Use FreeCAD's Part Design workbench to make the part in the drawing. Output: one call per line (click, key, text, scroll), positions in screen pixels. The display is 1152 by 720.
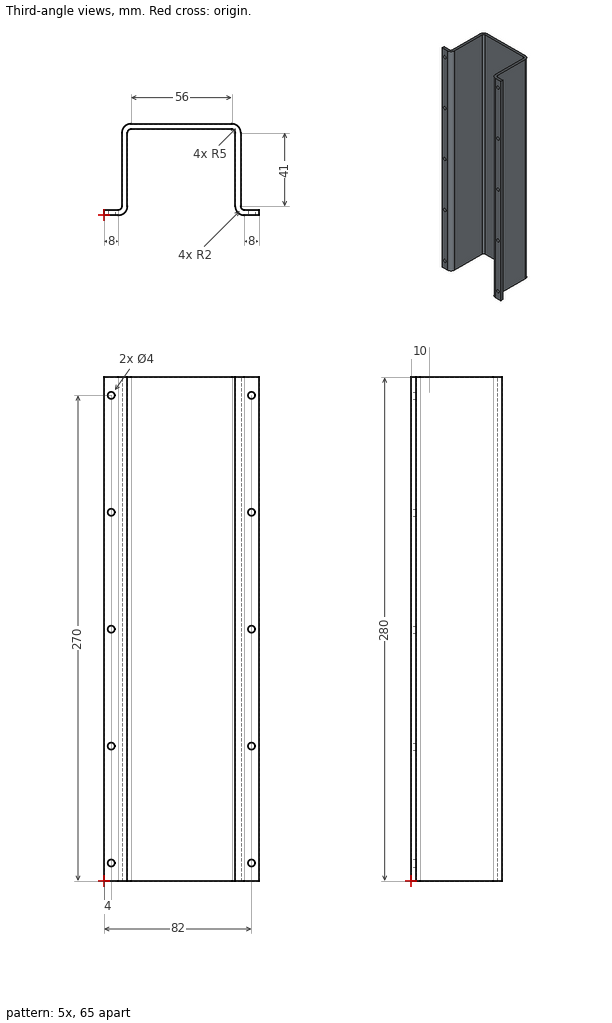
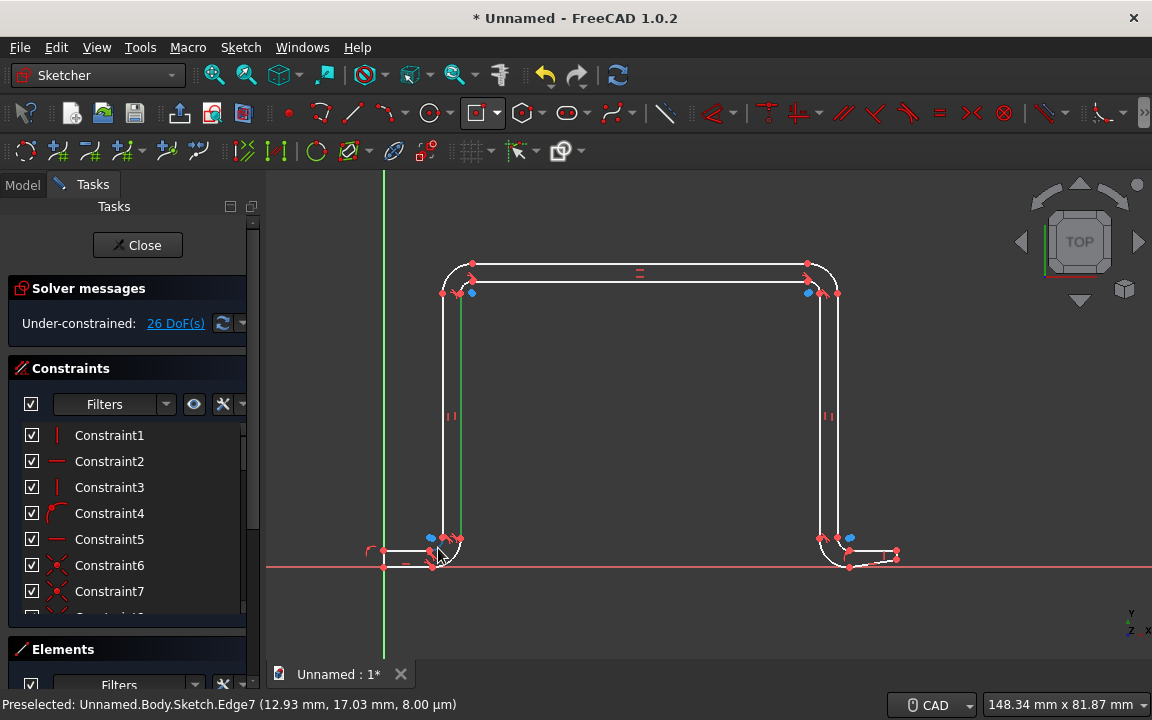
scroll(467, 283, up, 5)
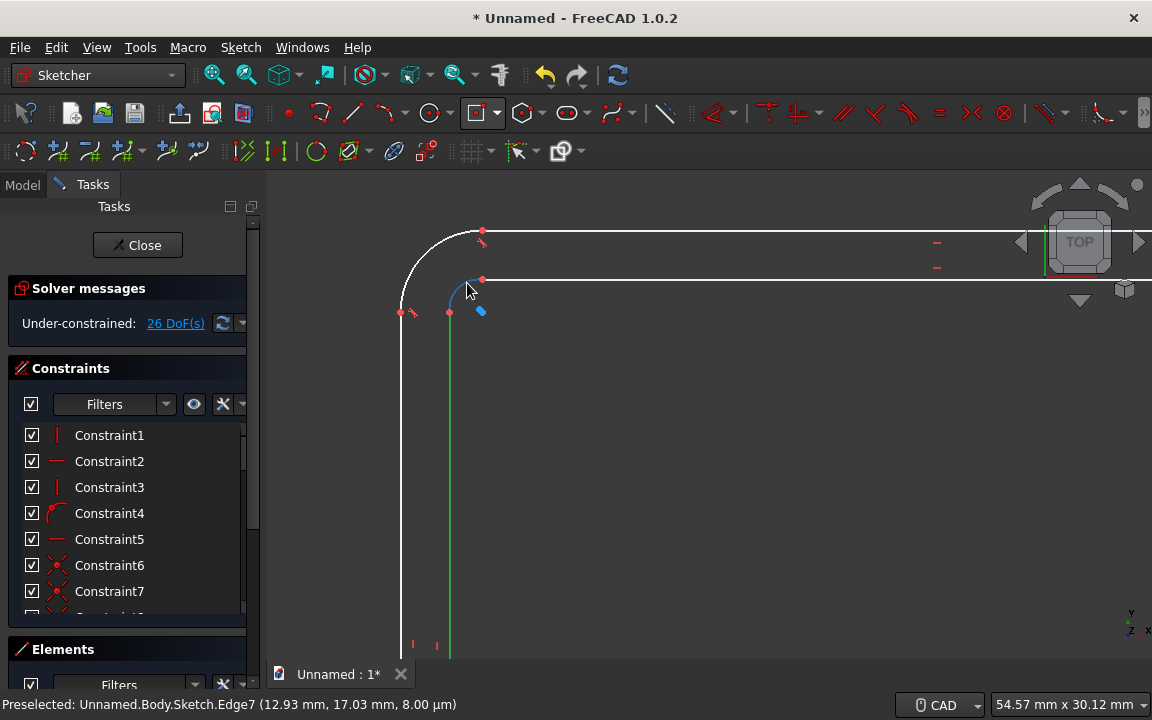
click(467, 282)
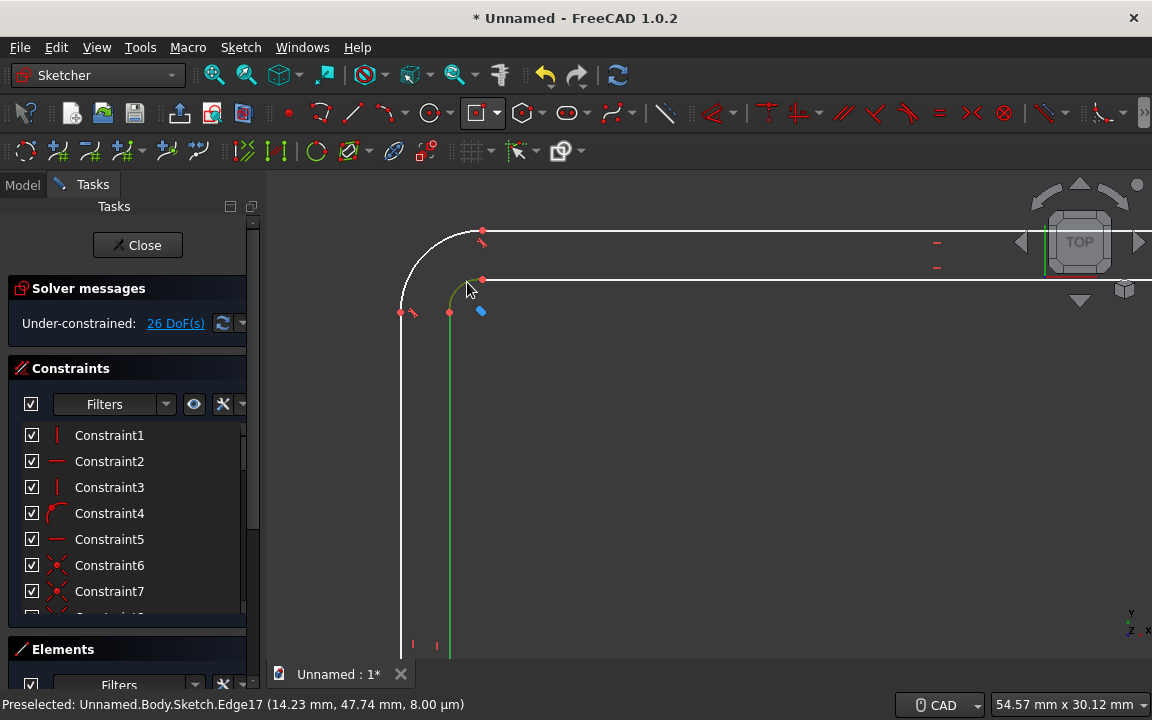
click(908, 114)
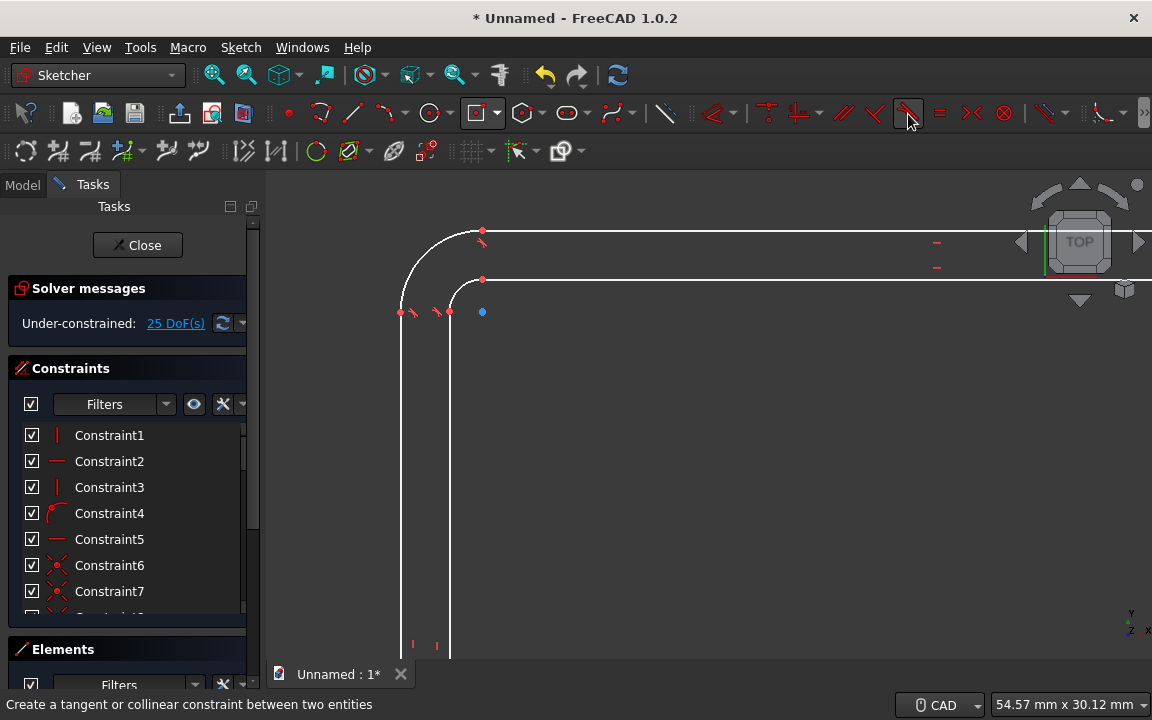
click(756, 280)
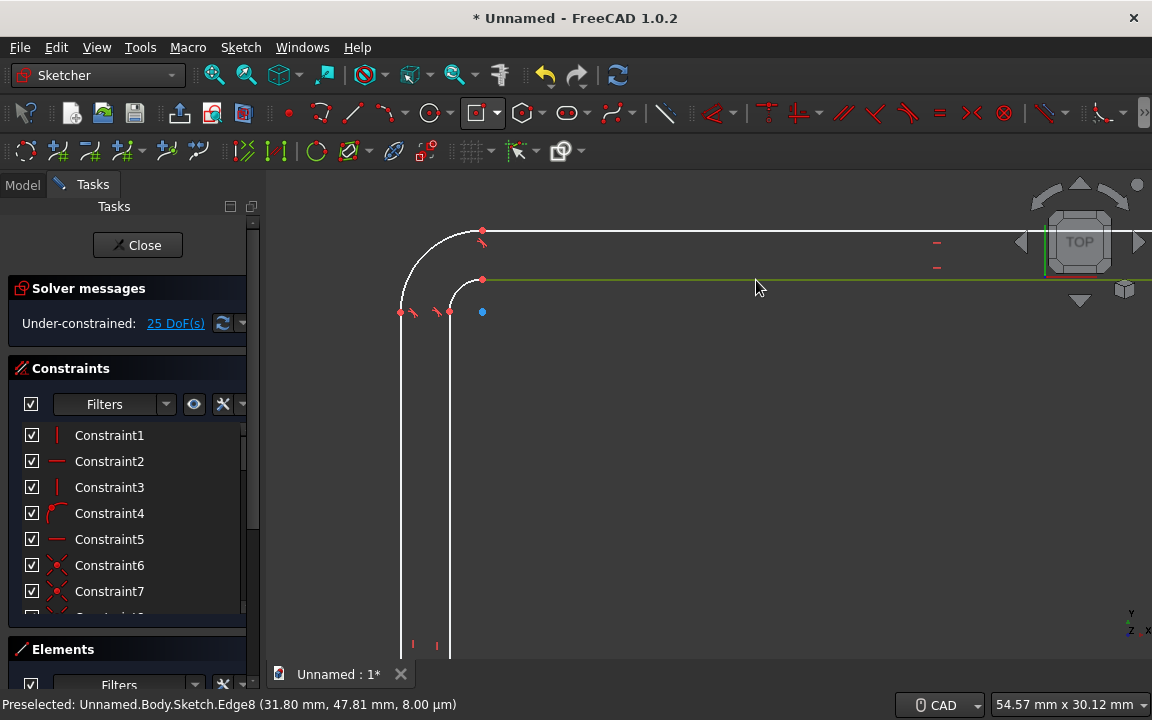
click(468, 283)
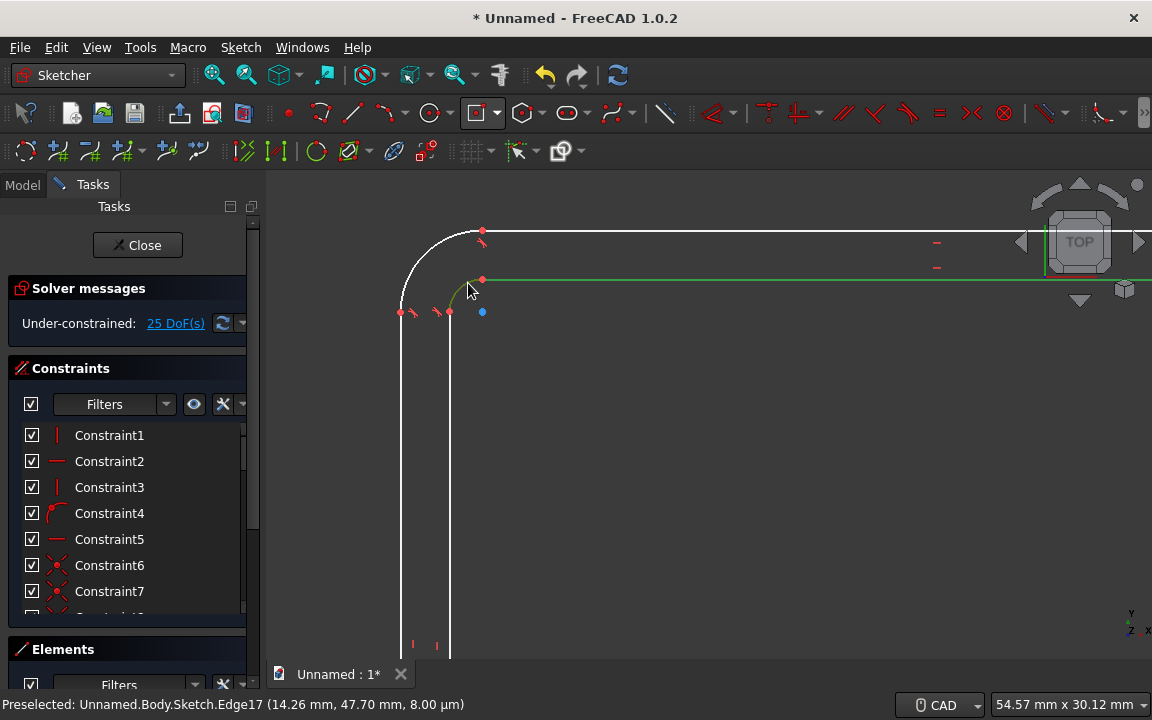
key(t)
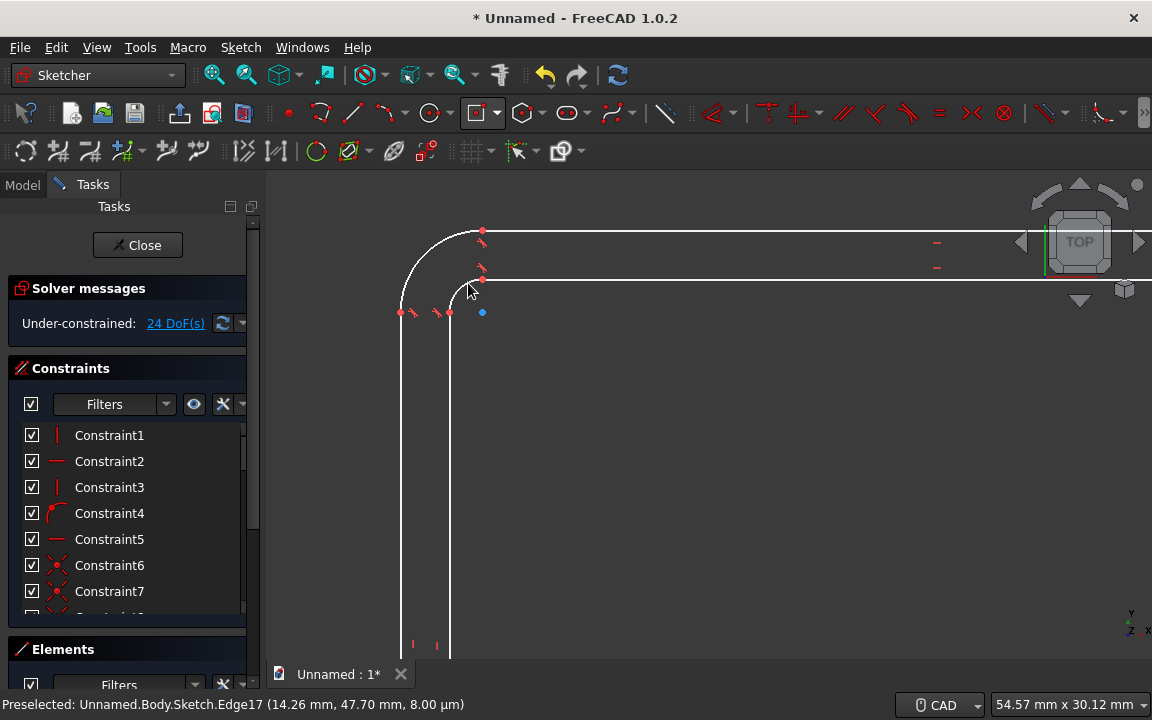
click(756, 280)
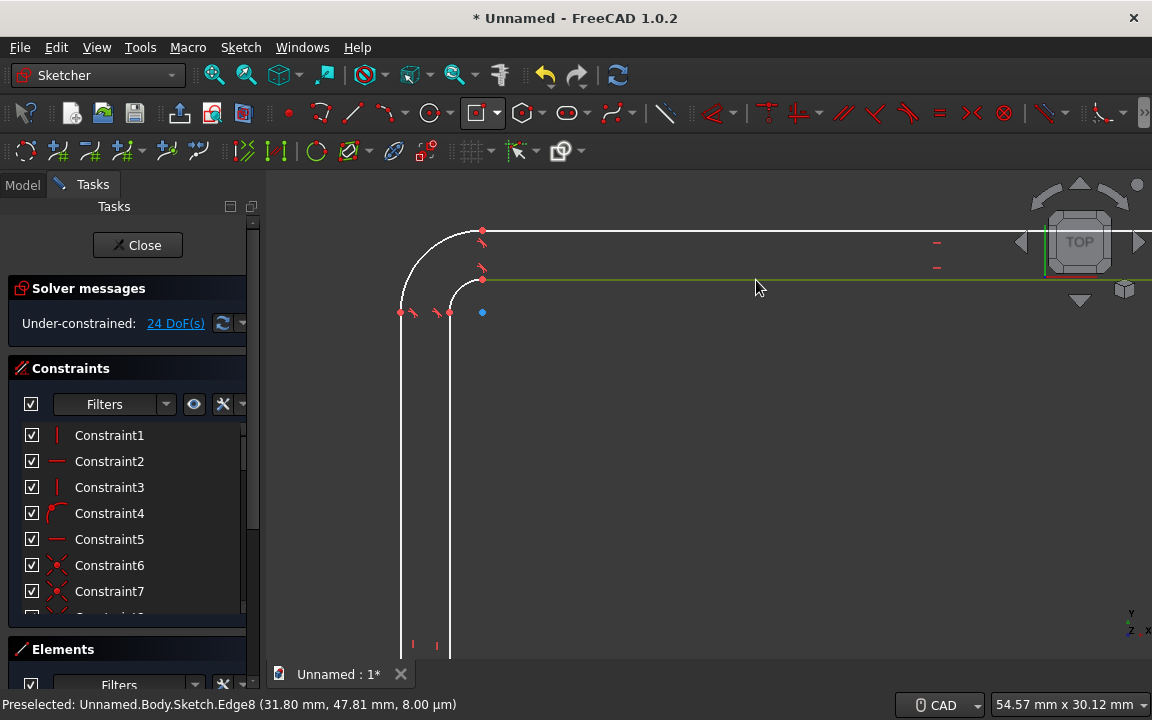
scroll(467, 282, down, 5)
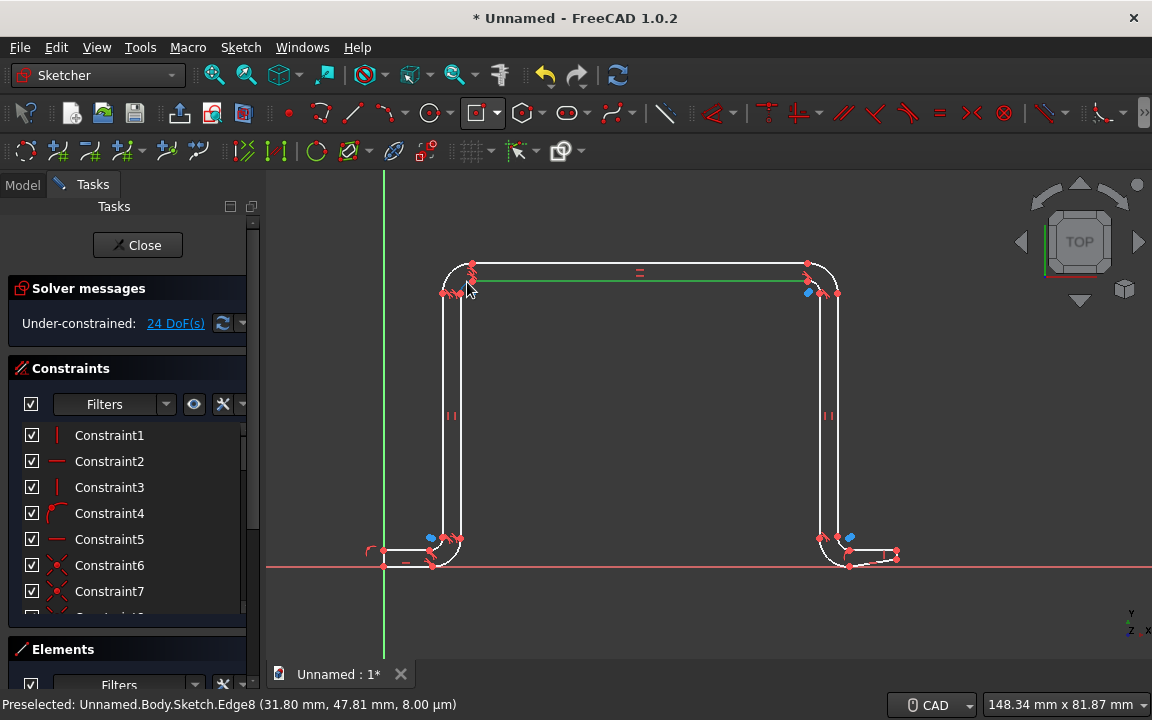
scroll(819, 288, up, 5)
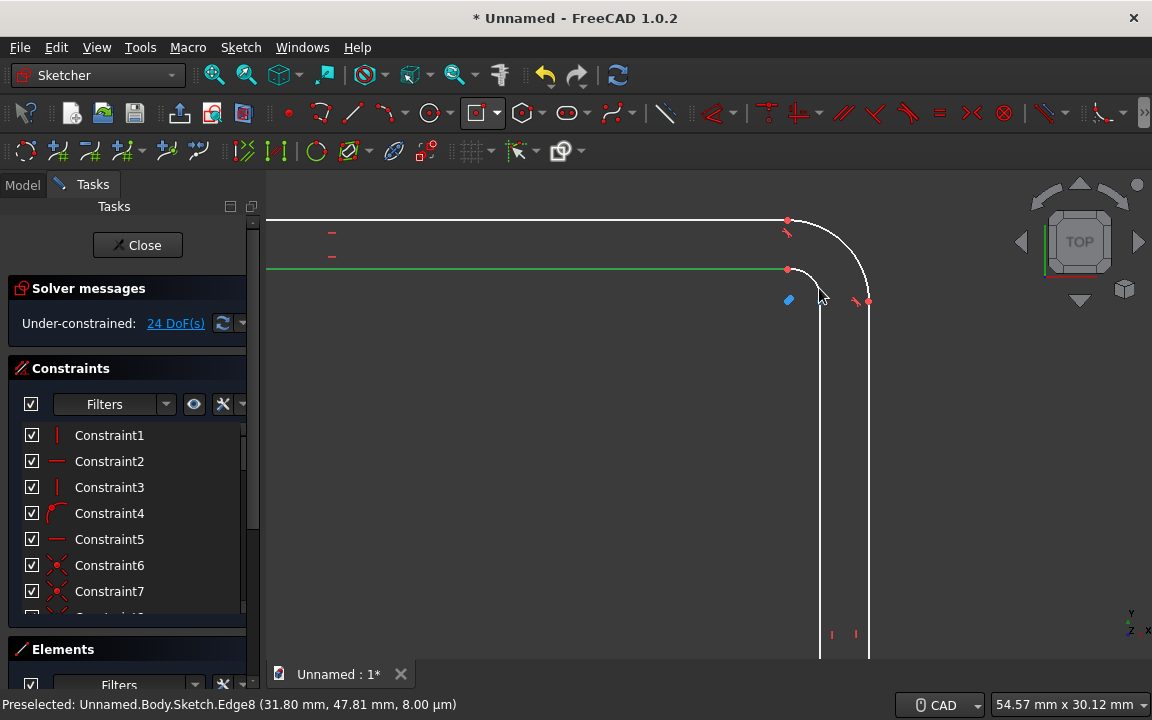
click(818, 286)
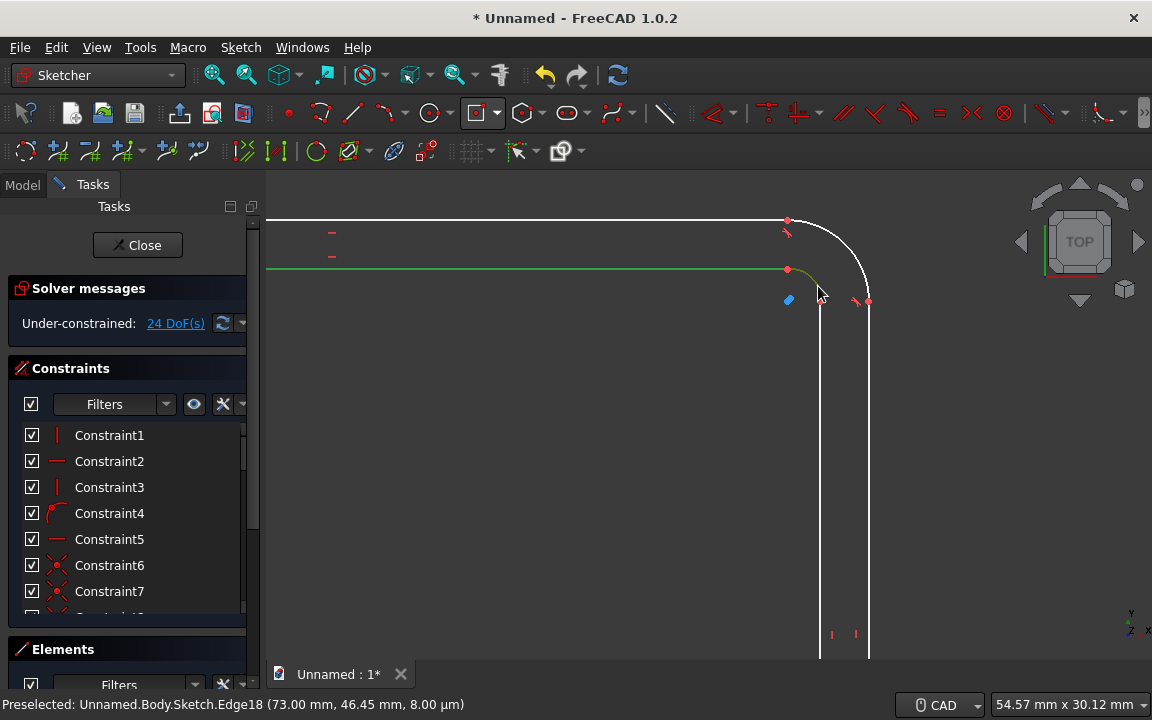
key(t)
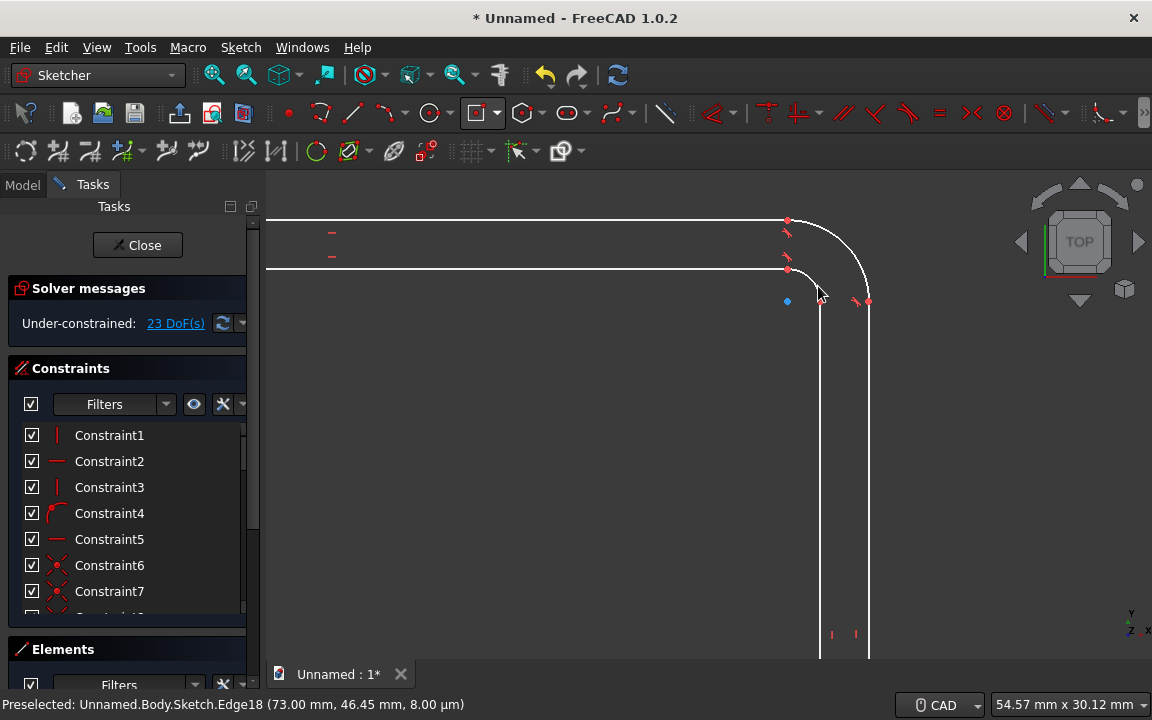
click(820, 502)